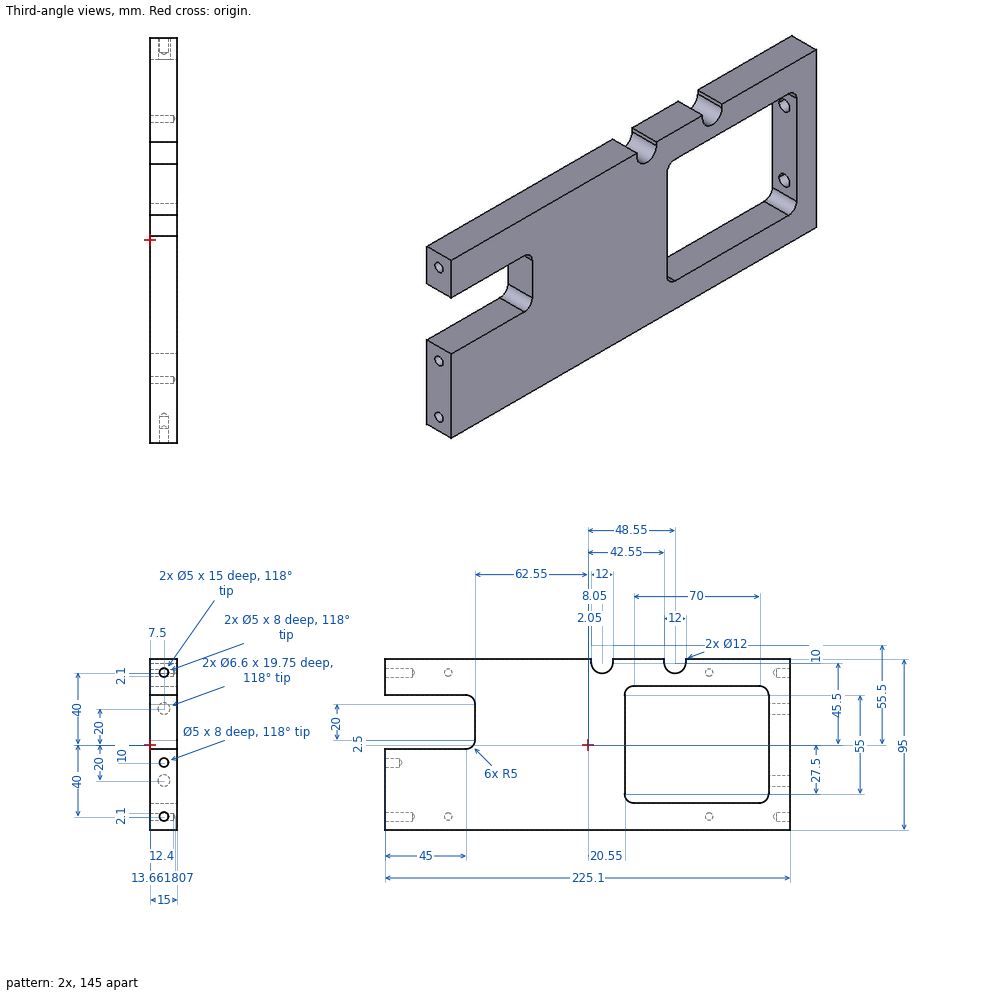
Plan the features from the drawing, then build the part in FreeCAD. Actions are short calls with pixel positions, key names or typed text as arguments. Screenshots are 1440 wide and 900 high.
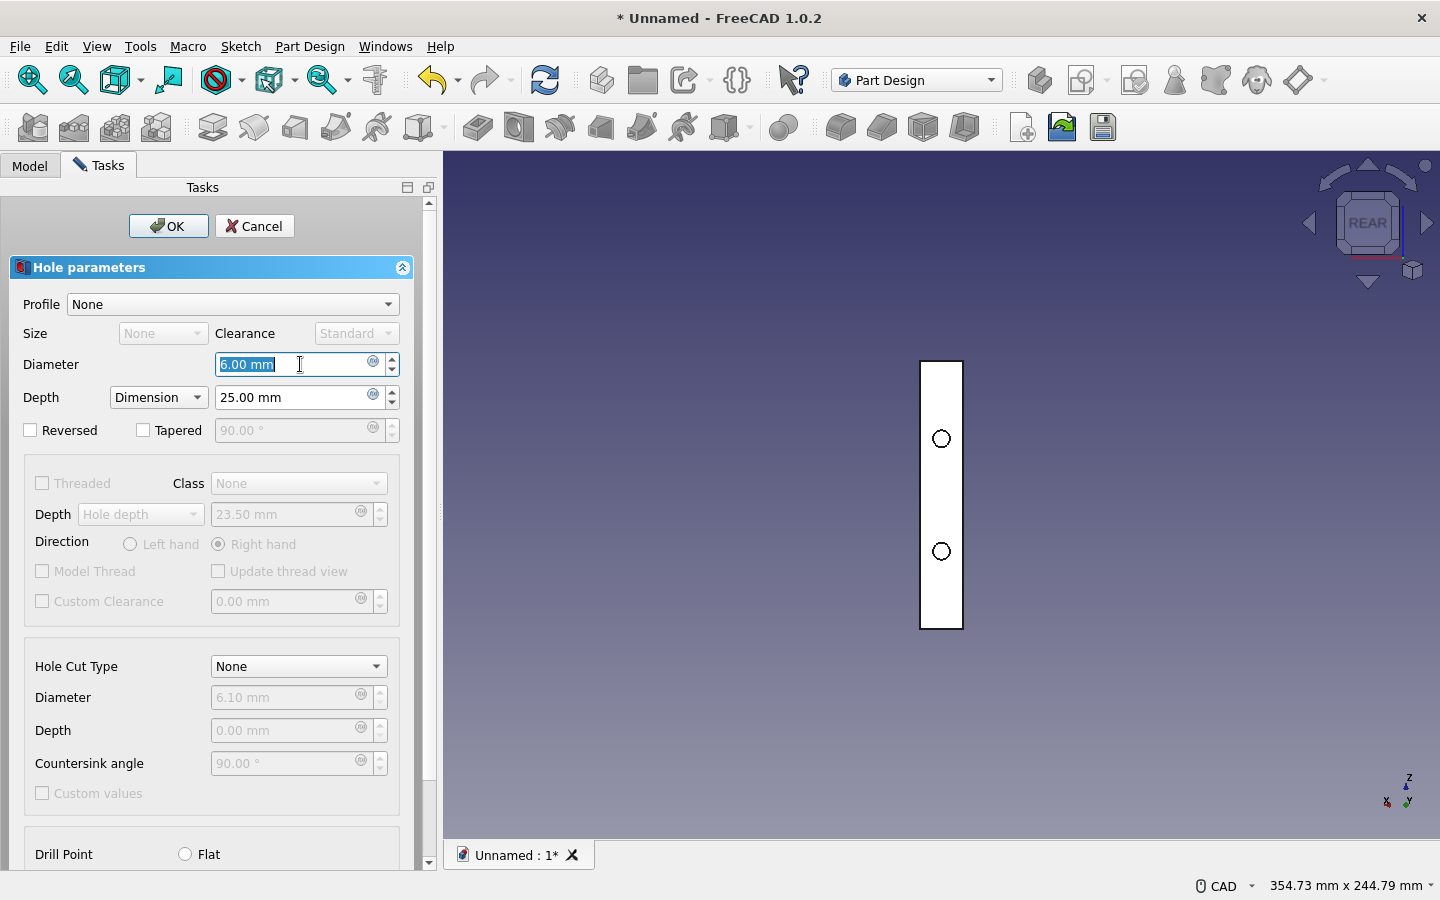
text(6.6)
key(Tab)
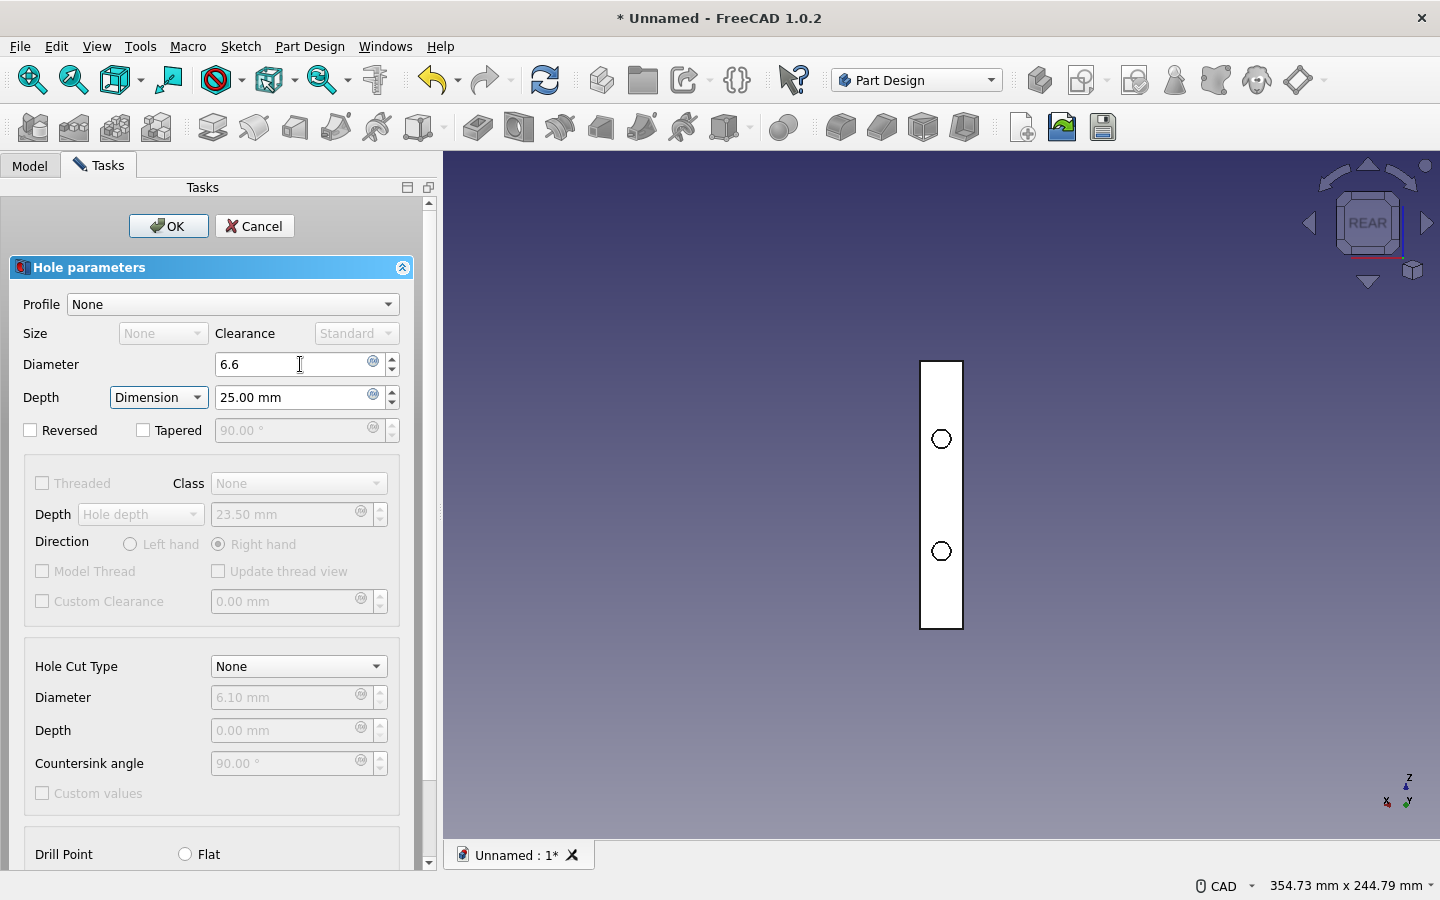
triple_click(300, 398)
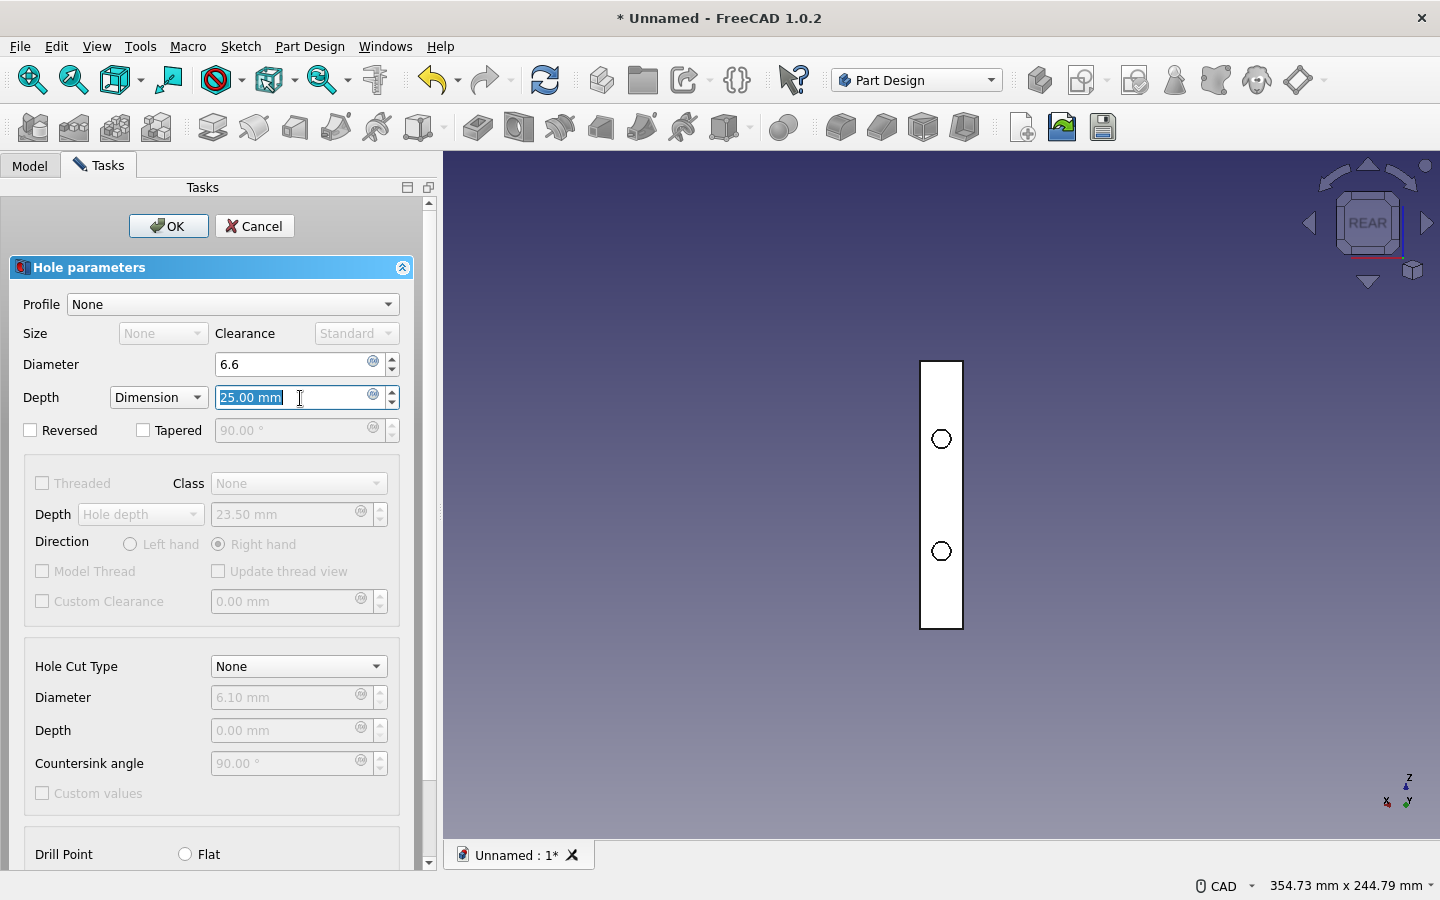
text(19.75)
key(Tab)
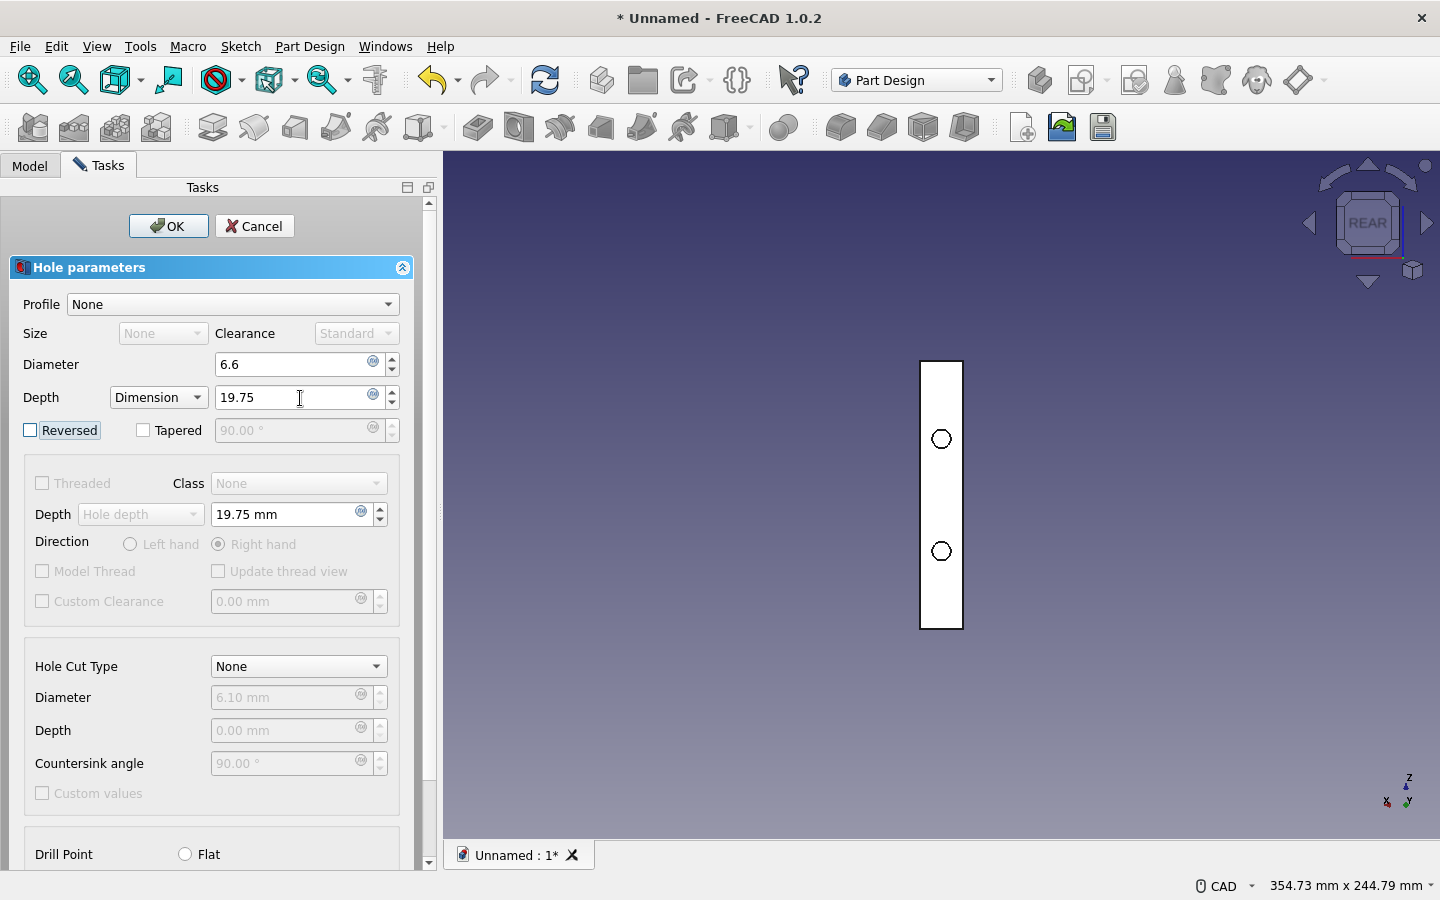
click(169, 226)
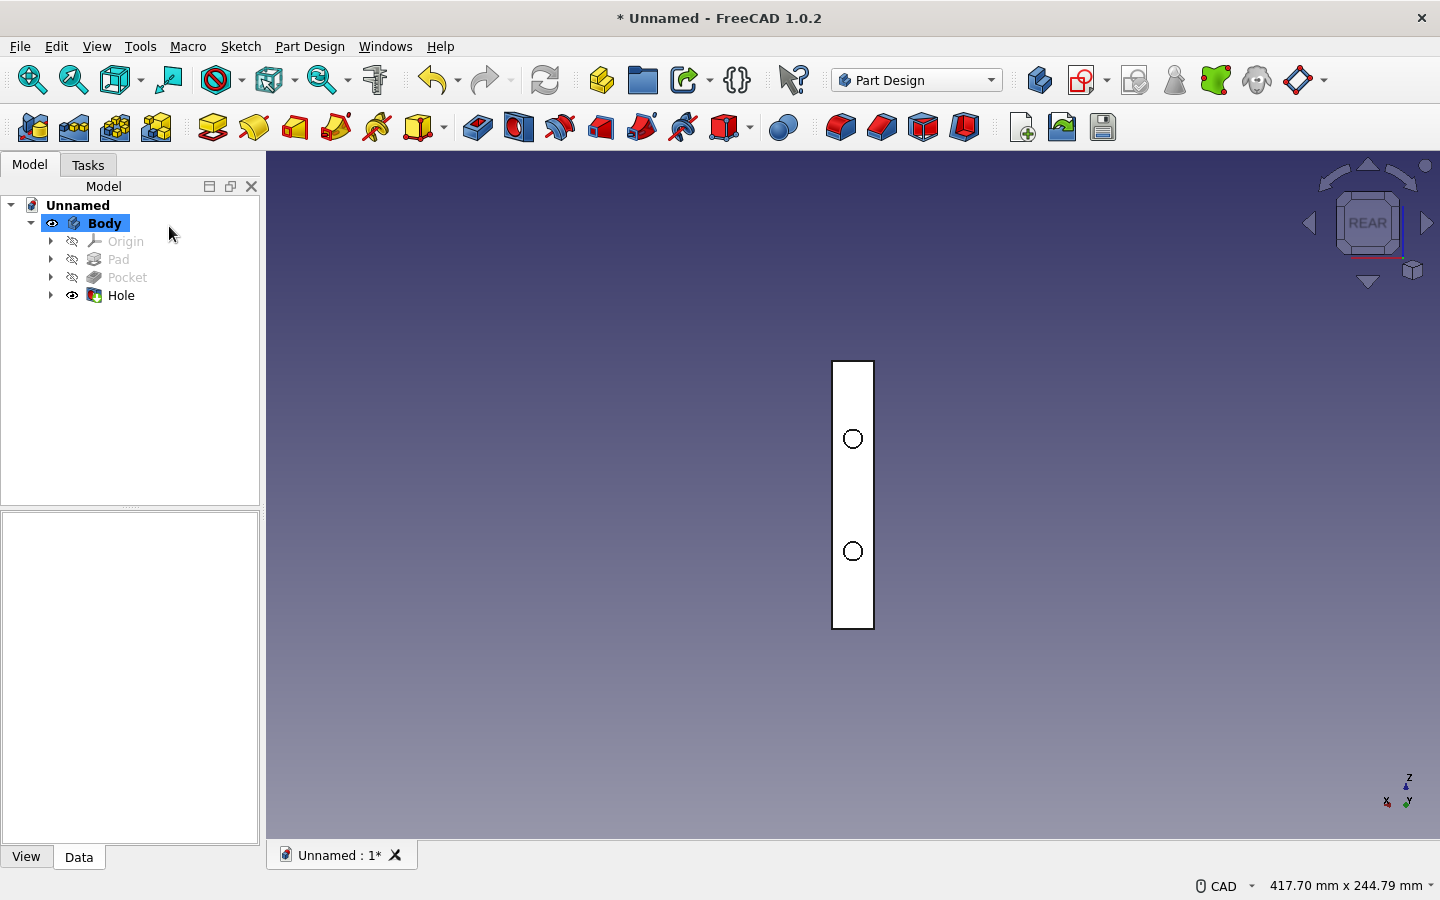
click(33, 80)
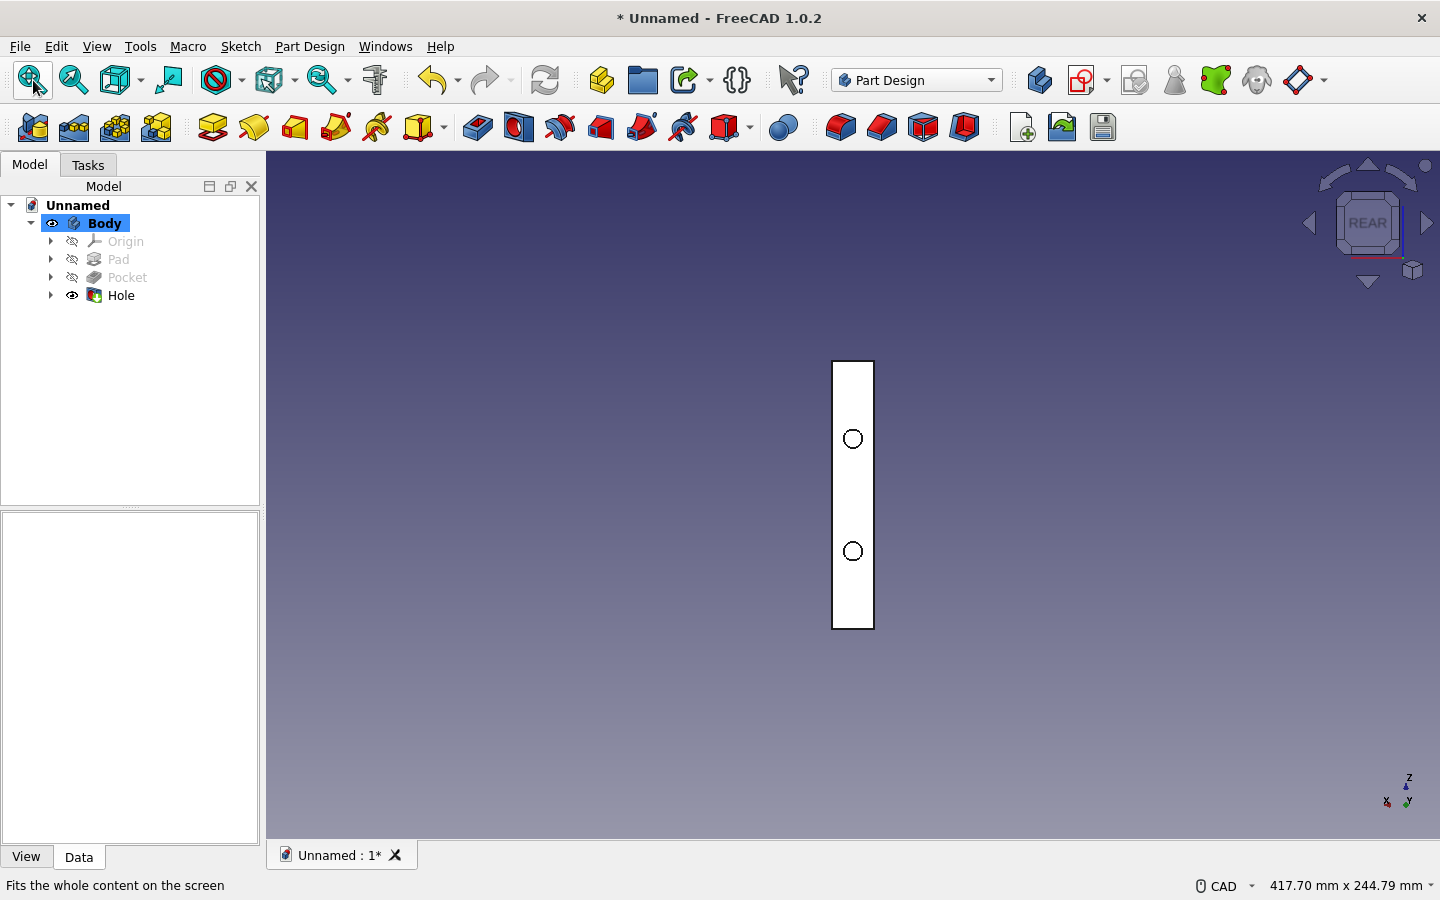
key(0)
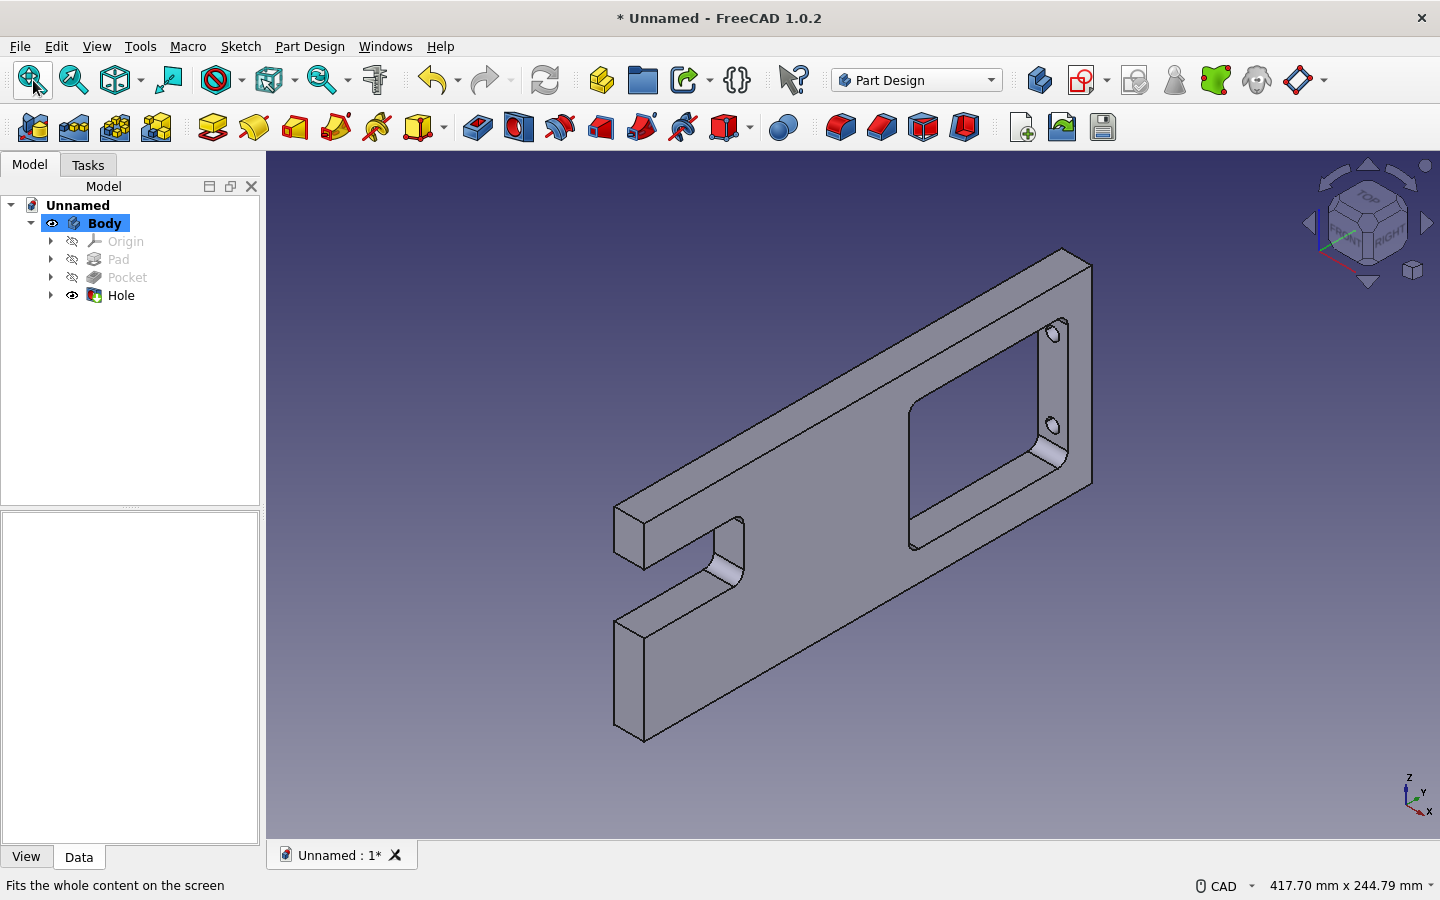
click(629, 710)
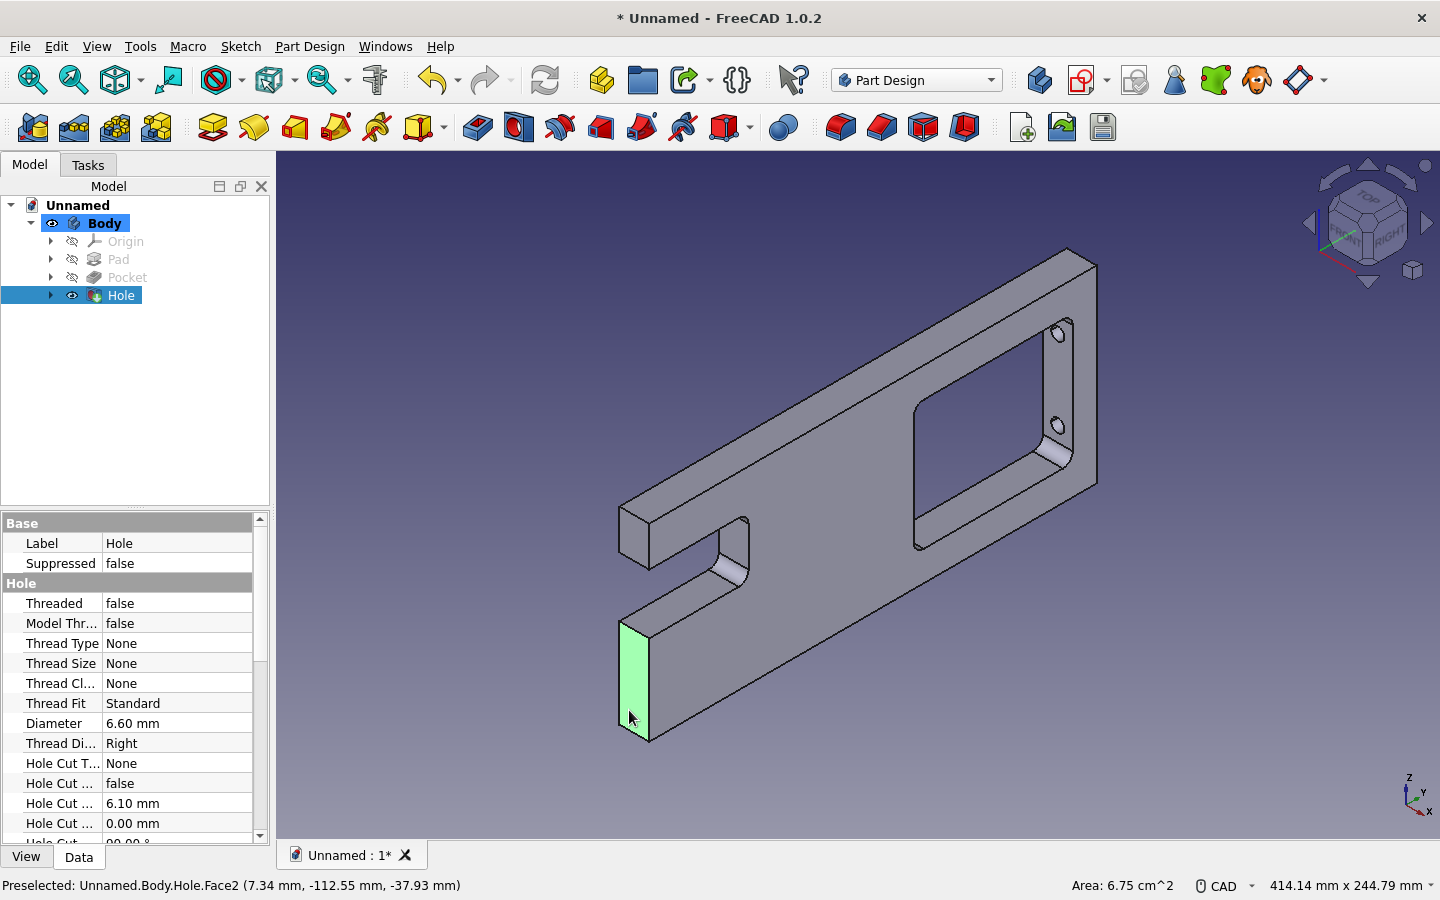
click(1080, 80)